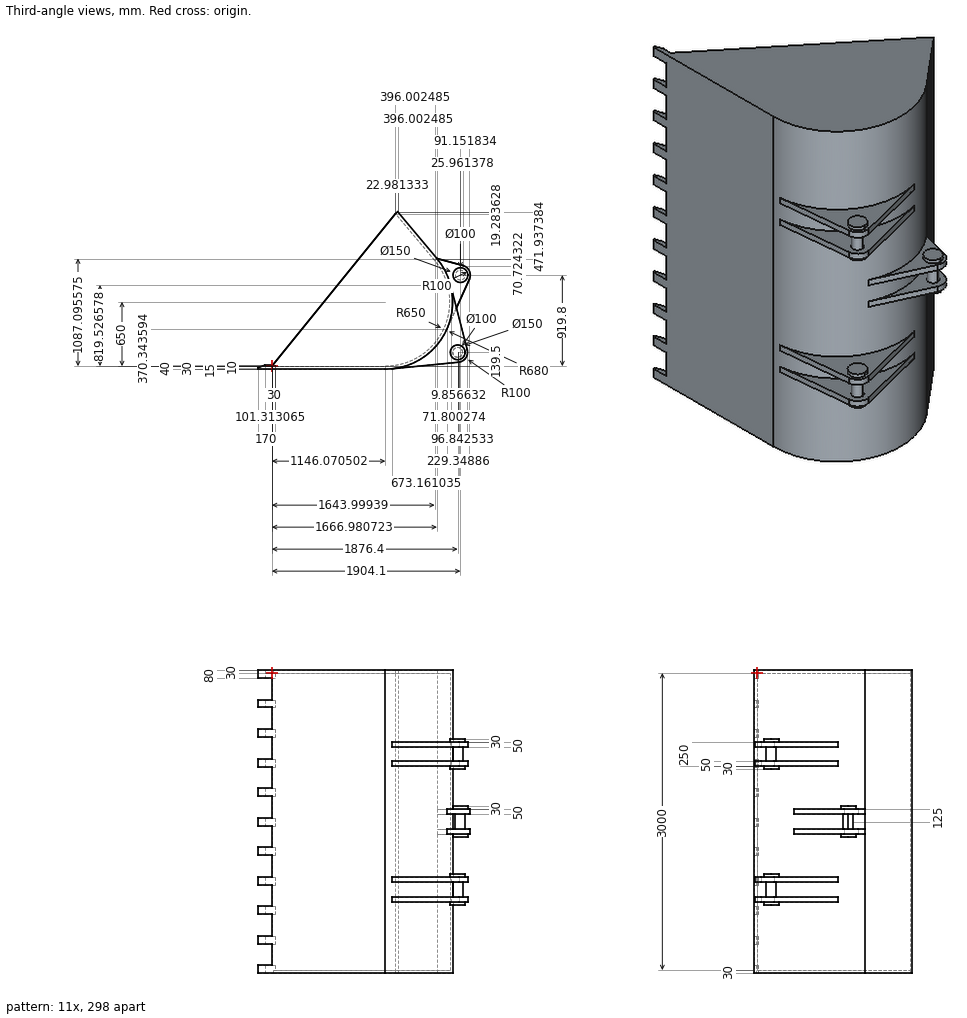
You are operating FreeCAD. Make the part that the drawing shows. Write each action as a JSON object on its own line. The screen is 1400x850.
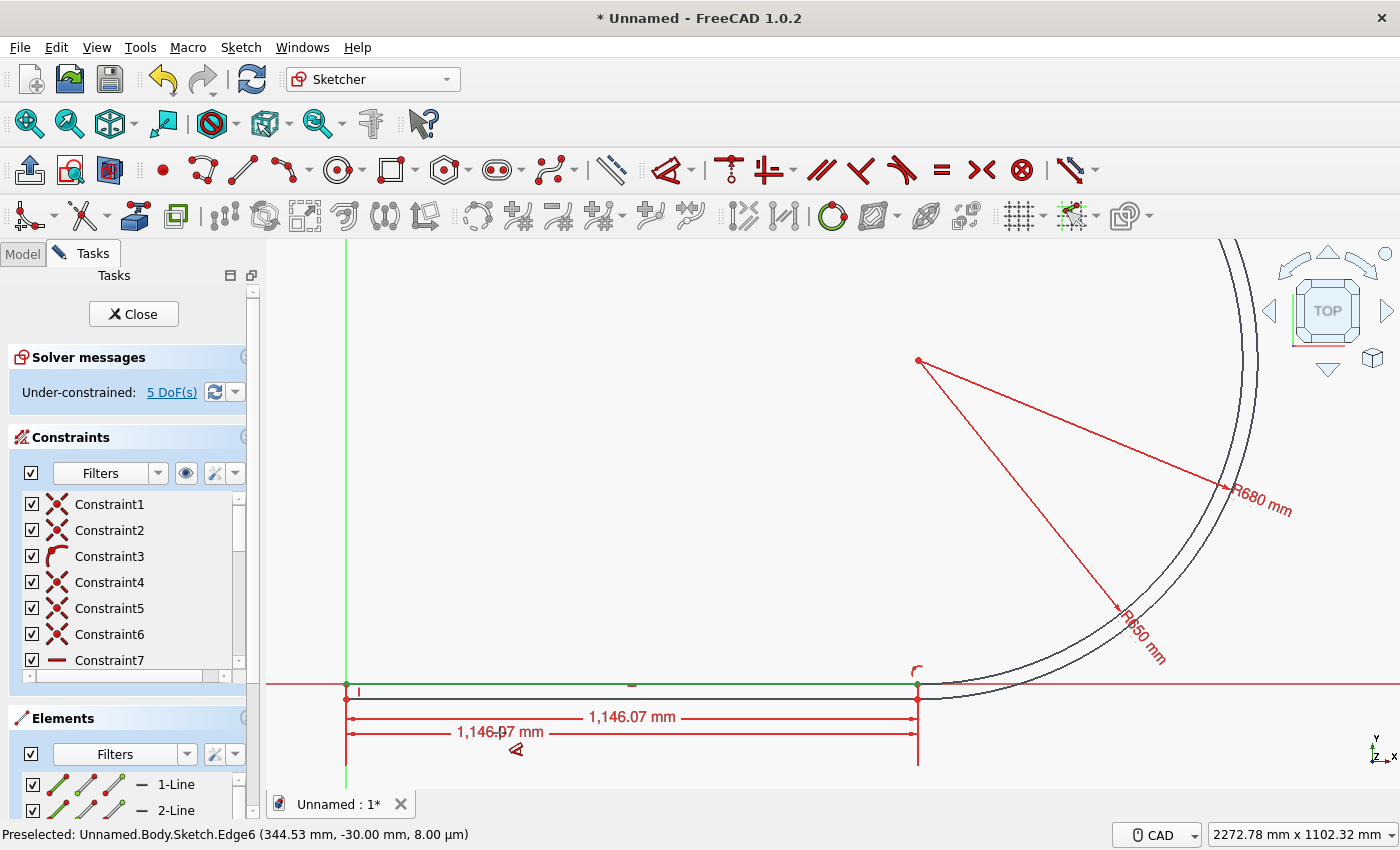
{"action": "scroll", "coordinate": [747, 686], "scroll_direction": "down", "scroll_amount": 4}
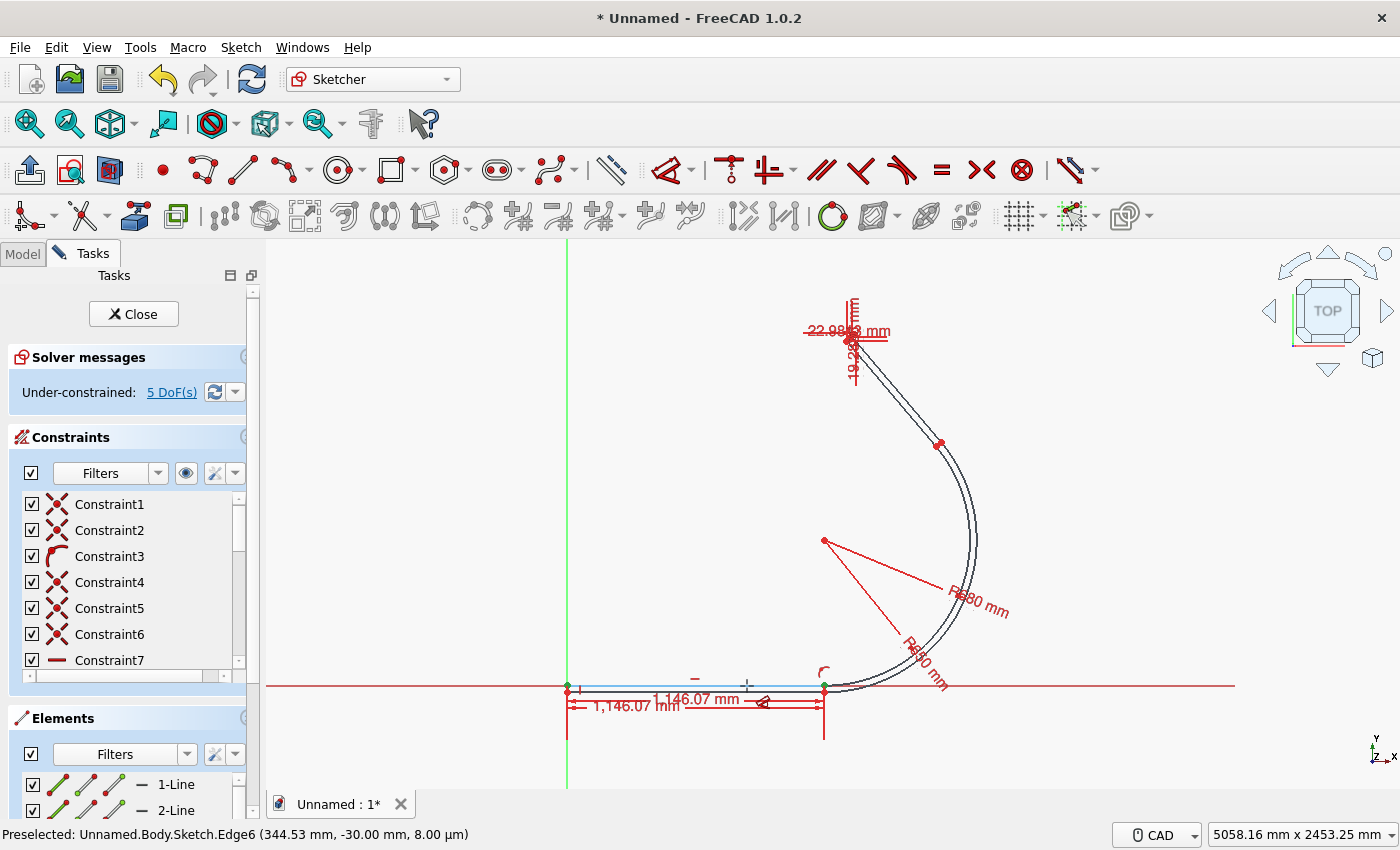
{"action": "scroll", "coordinate": [936, 447], "scroll_direction": "up", "scroll_amount": 3}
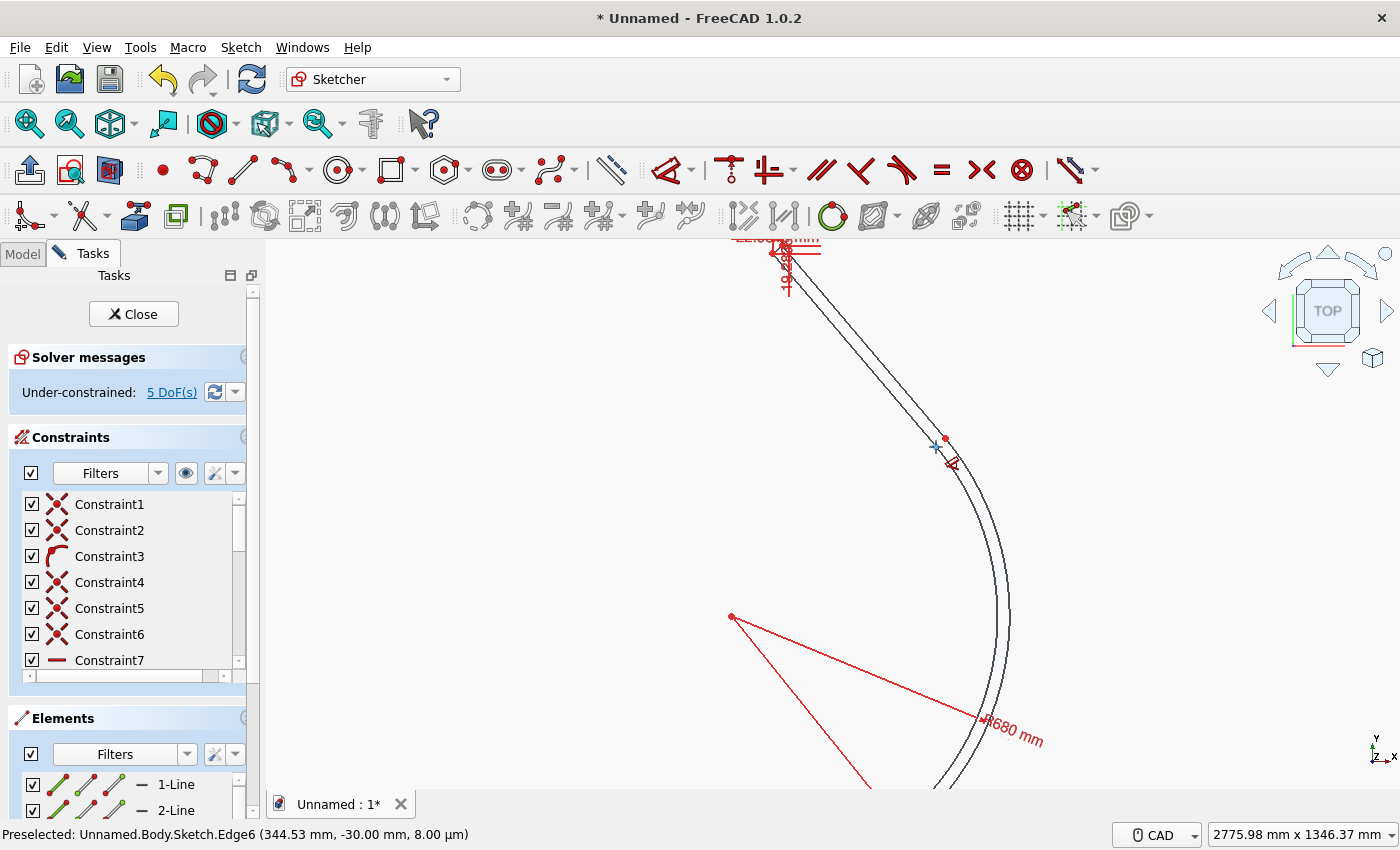
{"action": "left_click", "coordinate": [936, 446]}
{"action": "left_click", "coordinate": [615, 412]}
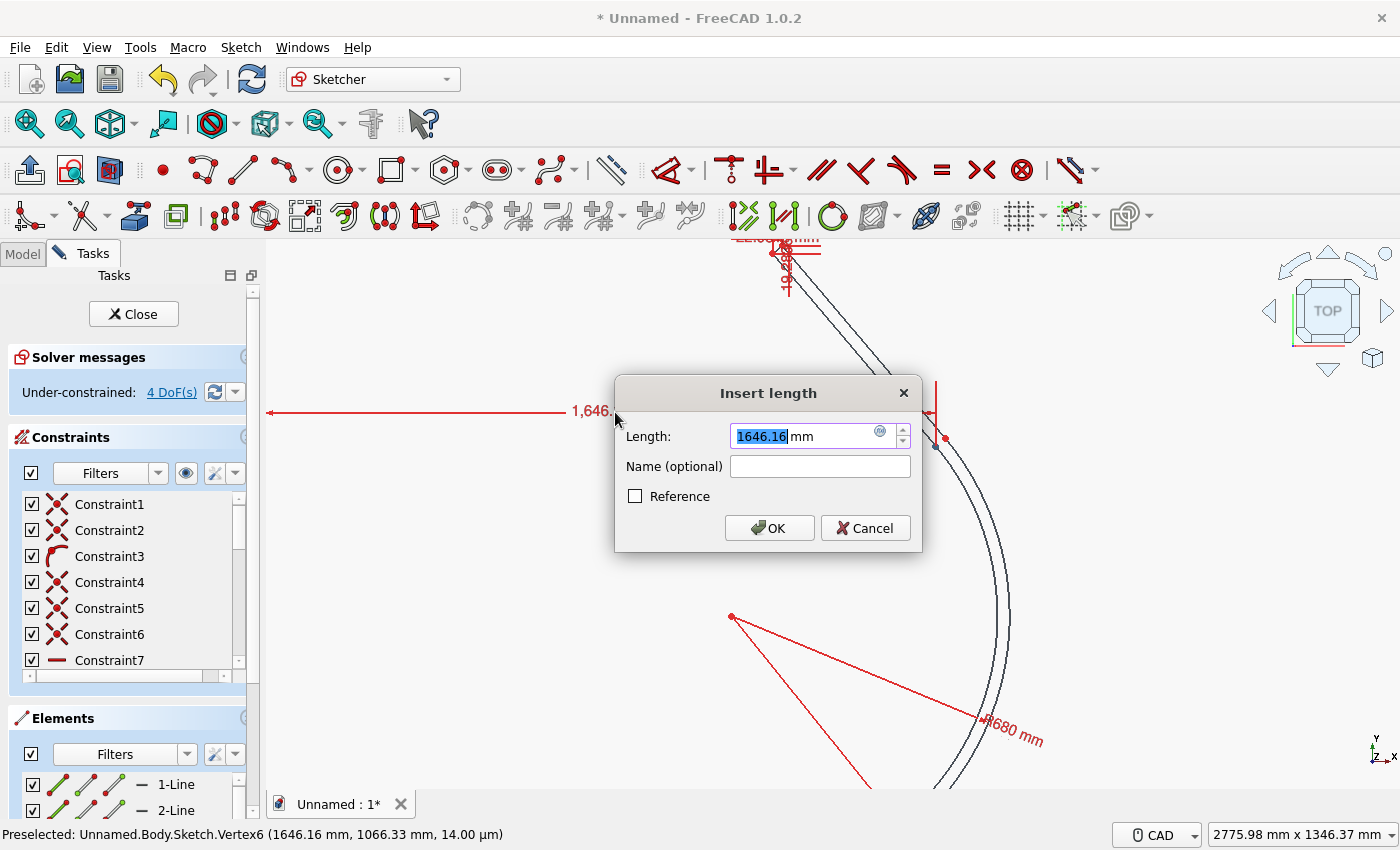
{"action": "type", "text": "1643.99939"}
{"action": "key", "text": "Return"}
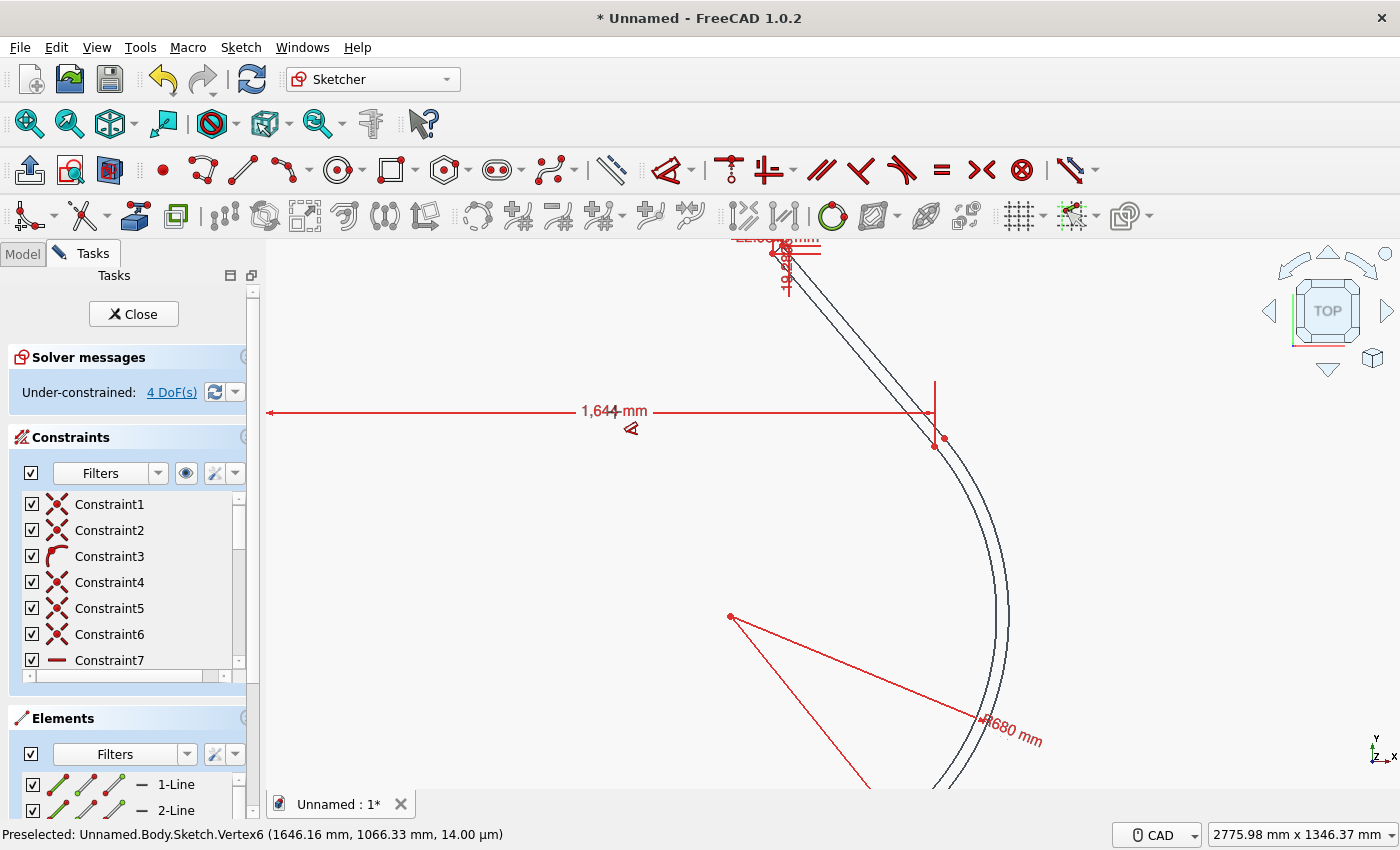
{"action": "left_click", "coordinate": [896, 381]}
{"action": "left_click", "coordinate": [863, 473]}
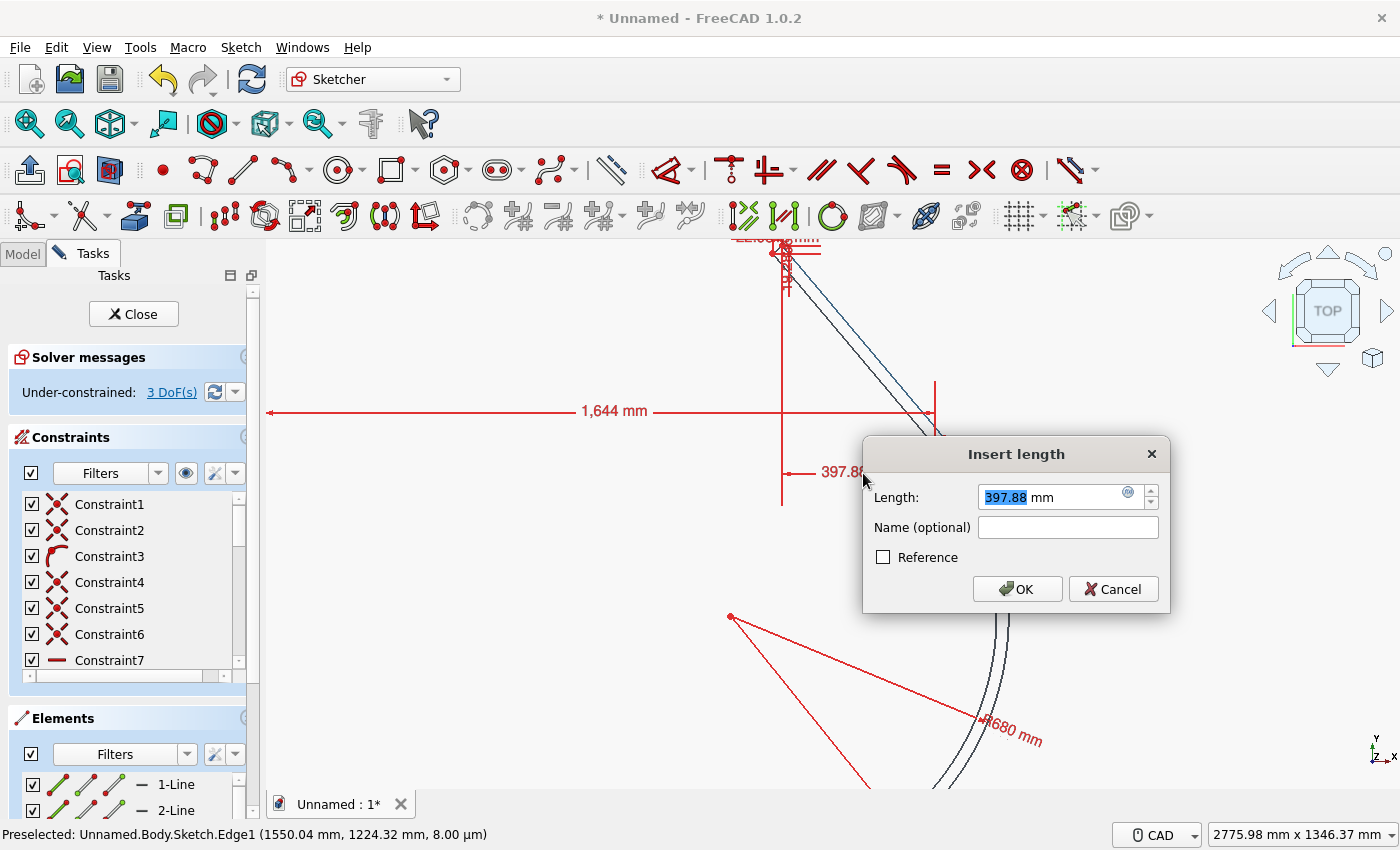
{"action": "type", "text": "396.002485"}
{"action": "key", "text": "Return"}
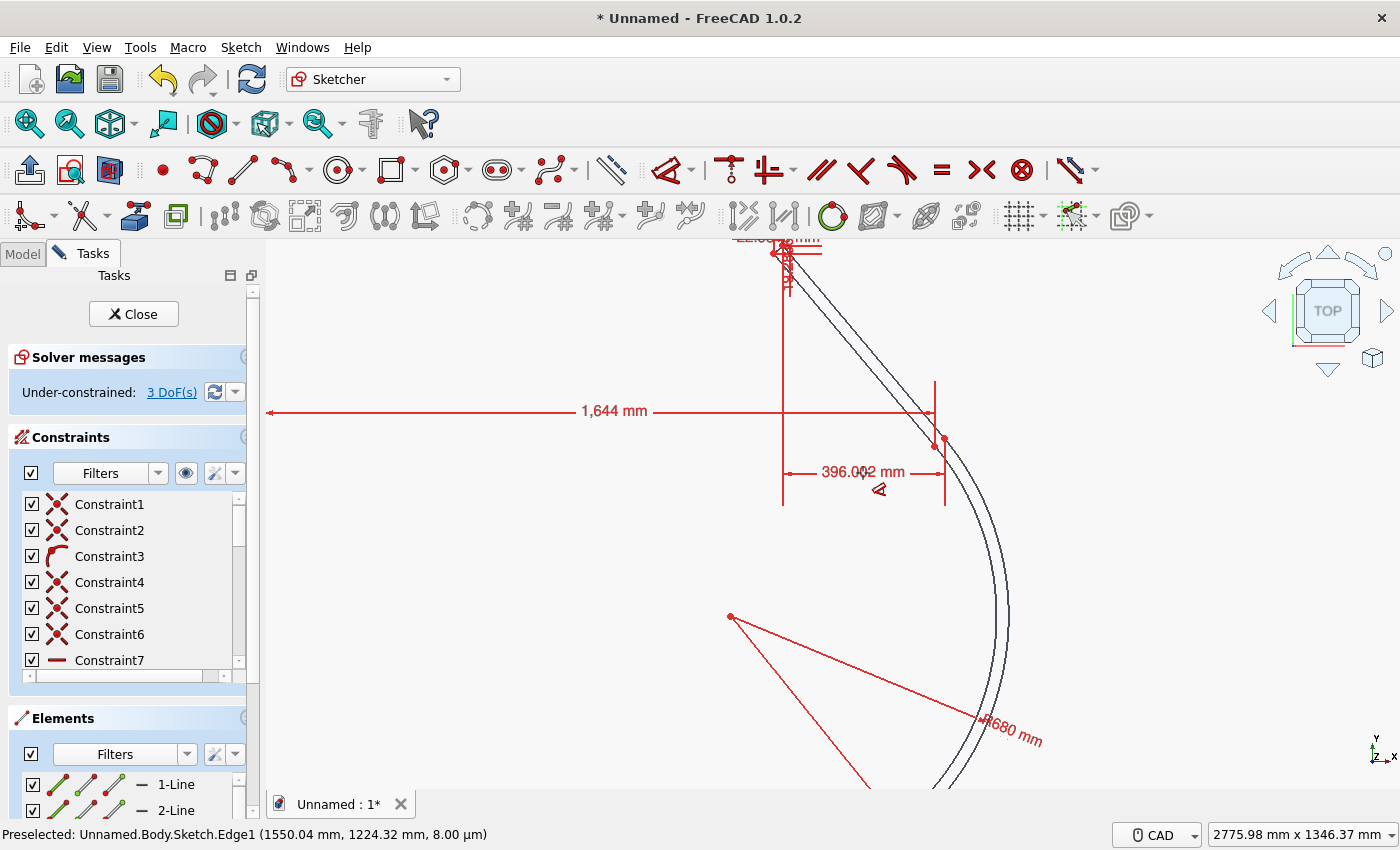
{"action": "left_click", "coordinate": [896, 381]}
{"action": "left_click", "coordinate": [979, 353]}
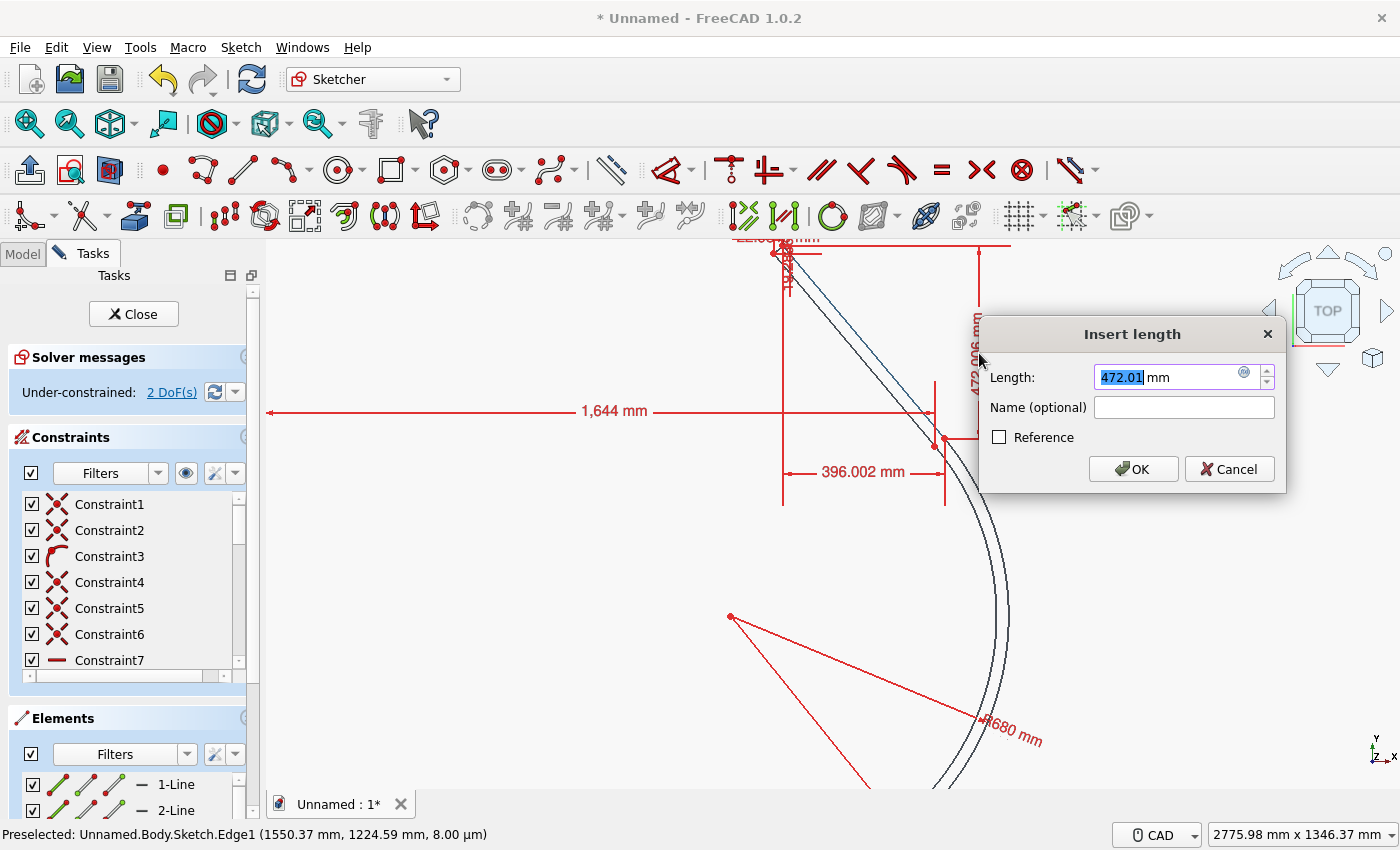
{"action": "type", "text": "471.937384"}
{"action": "key", "text": "Return"}